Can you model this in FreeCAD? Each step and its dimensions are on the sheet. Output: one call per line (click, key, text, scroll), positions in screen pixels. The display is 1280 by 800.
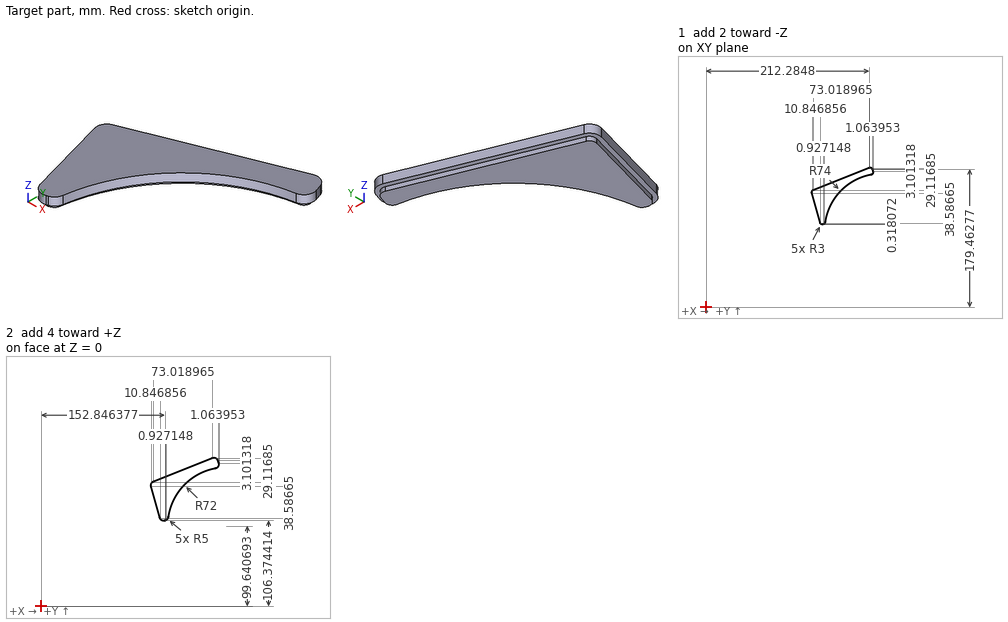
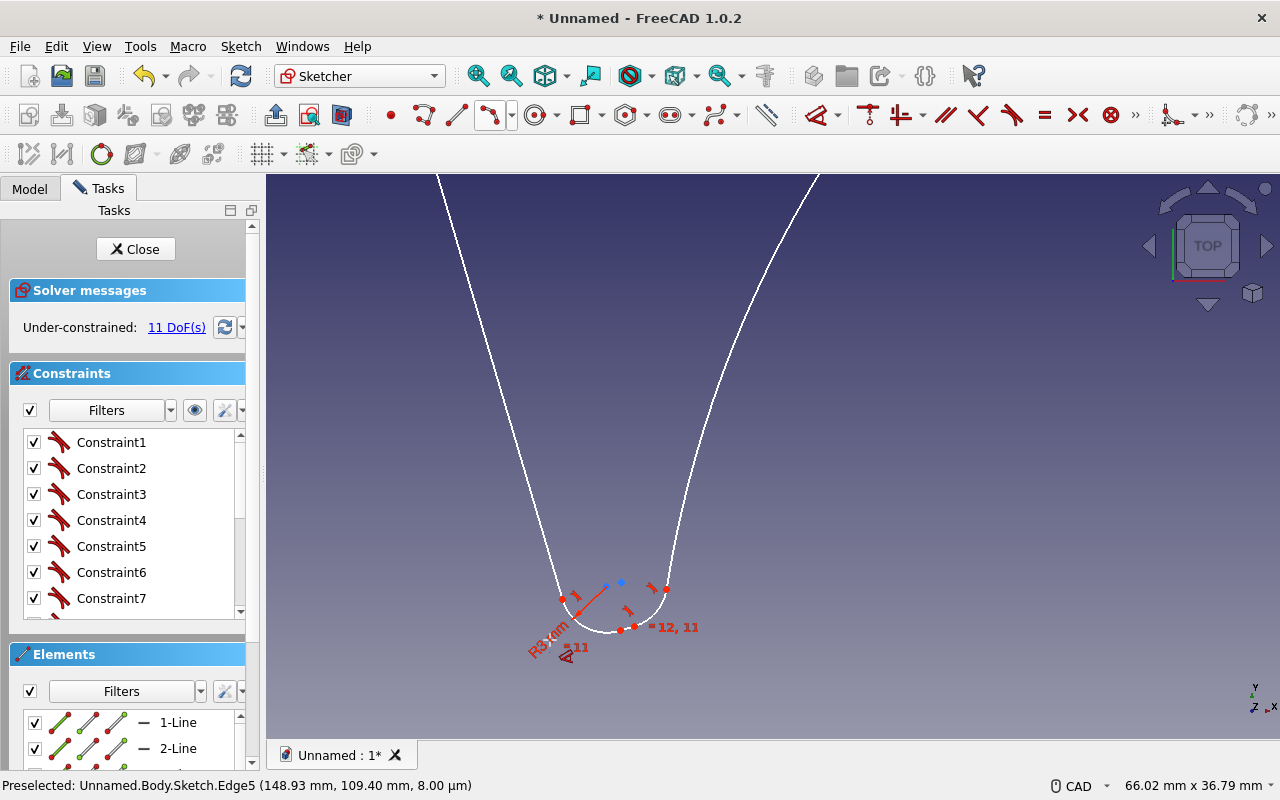
click(744, 321)
click(715, 308)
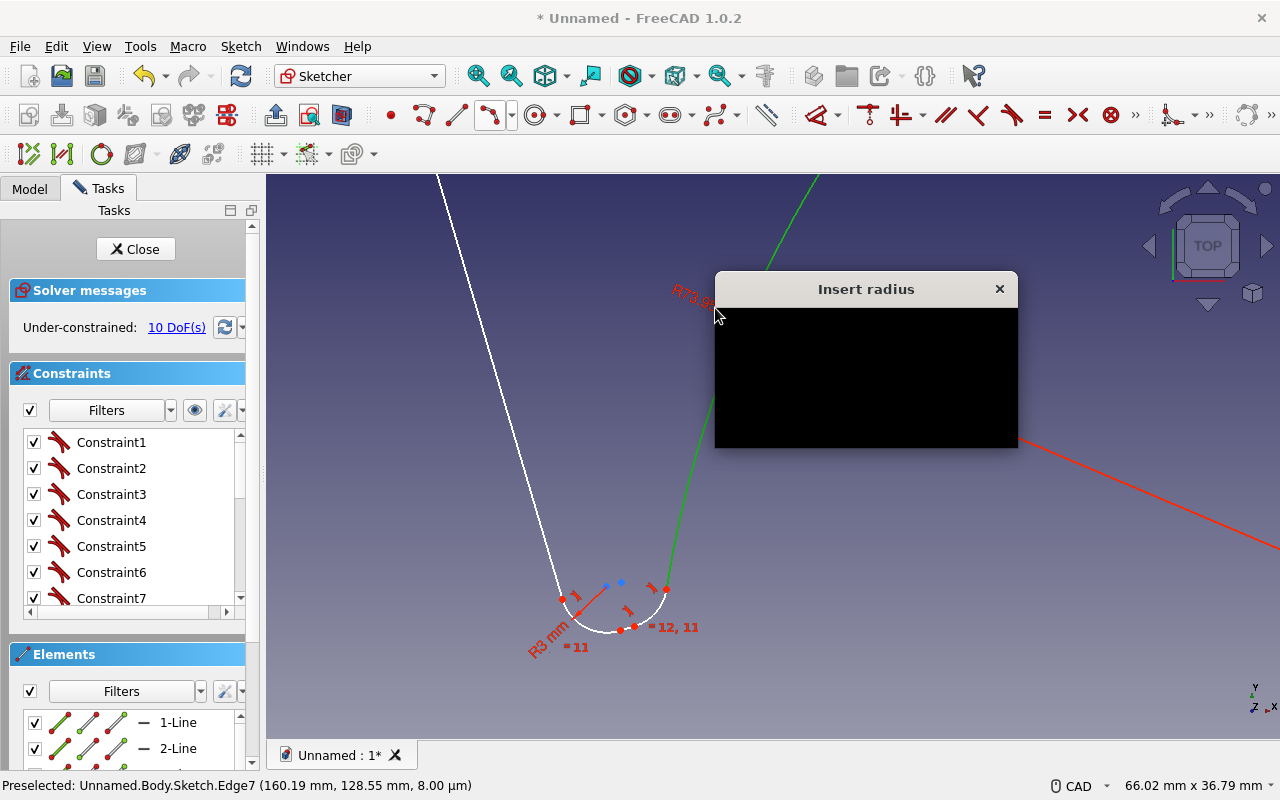
text(74)
key(Return)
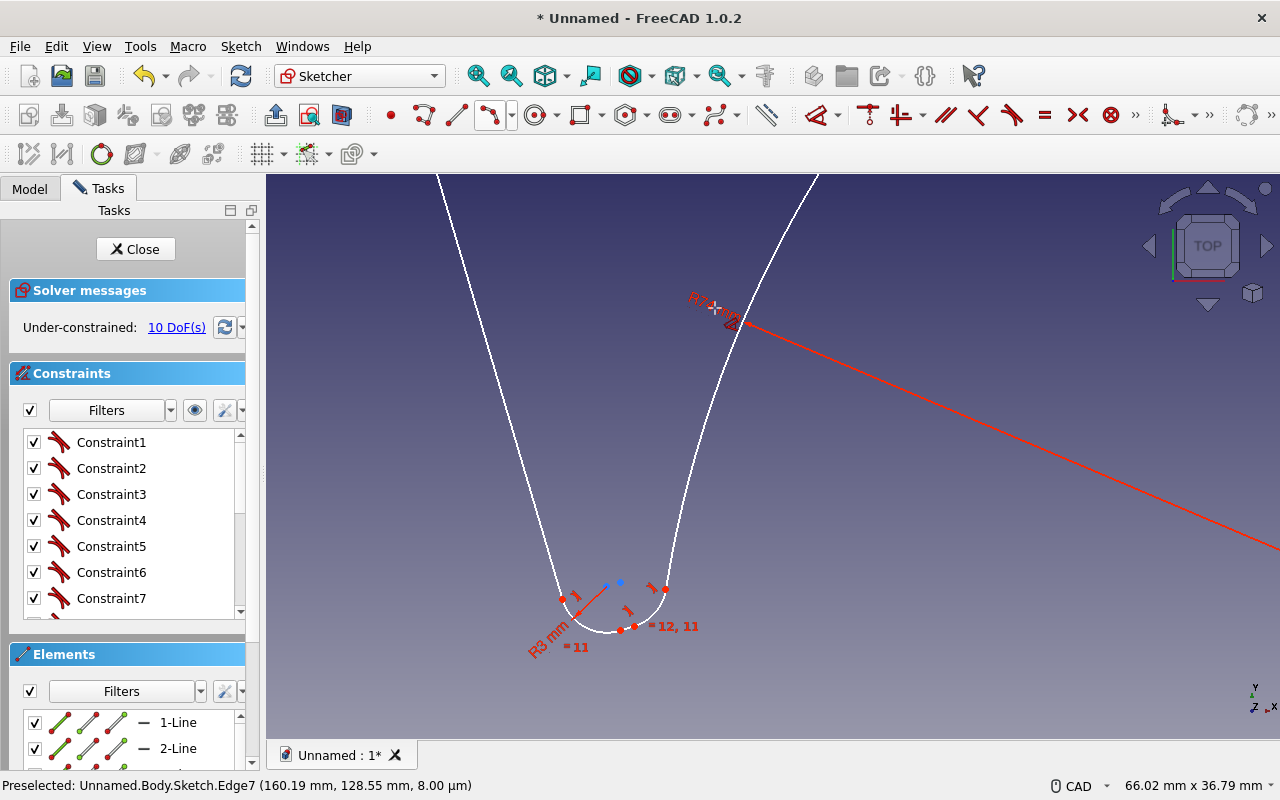
scroll(574, 621, down, 6)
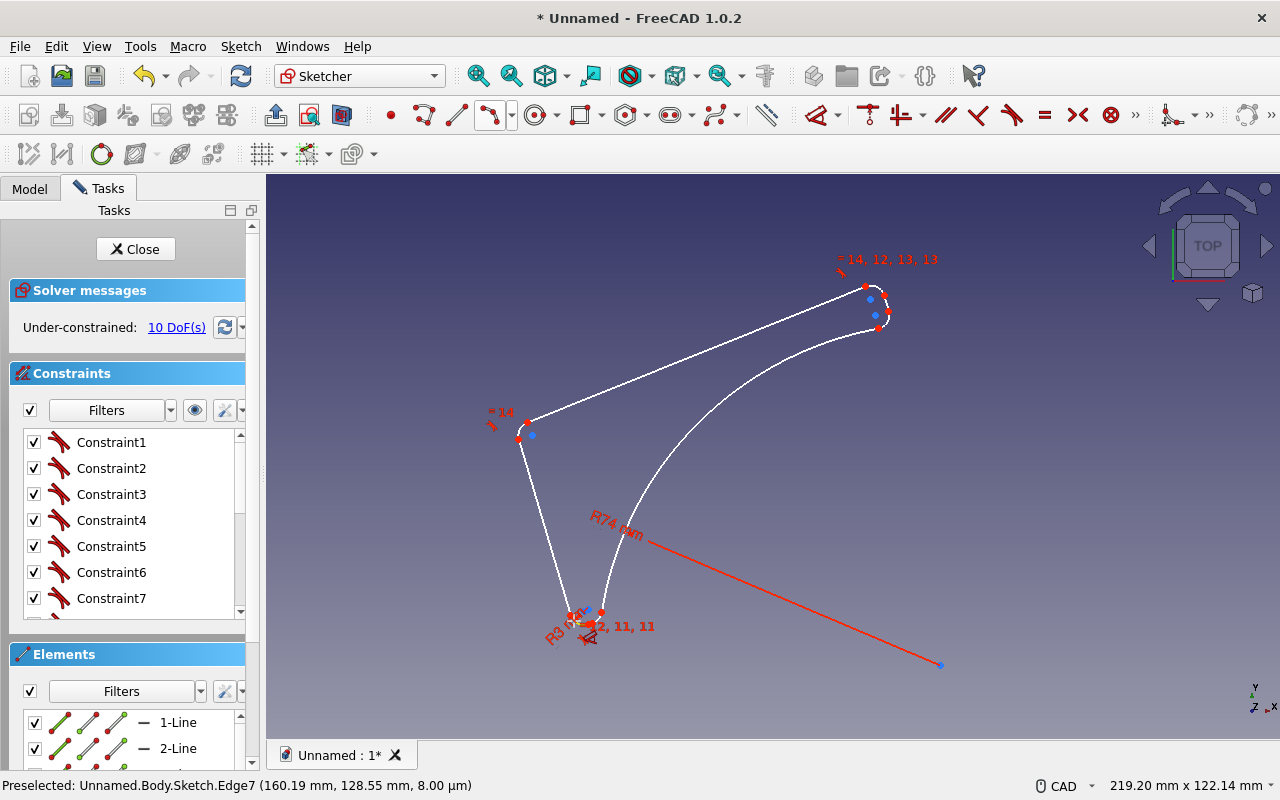
click(866, 287)
click(580, 253)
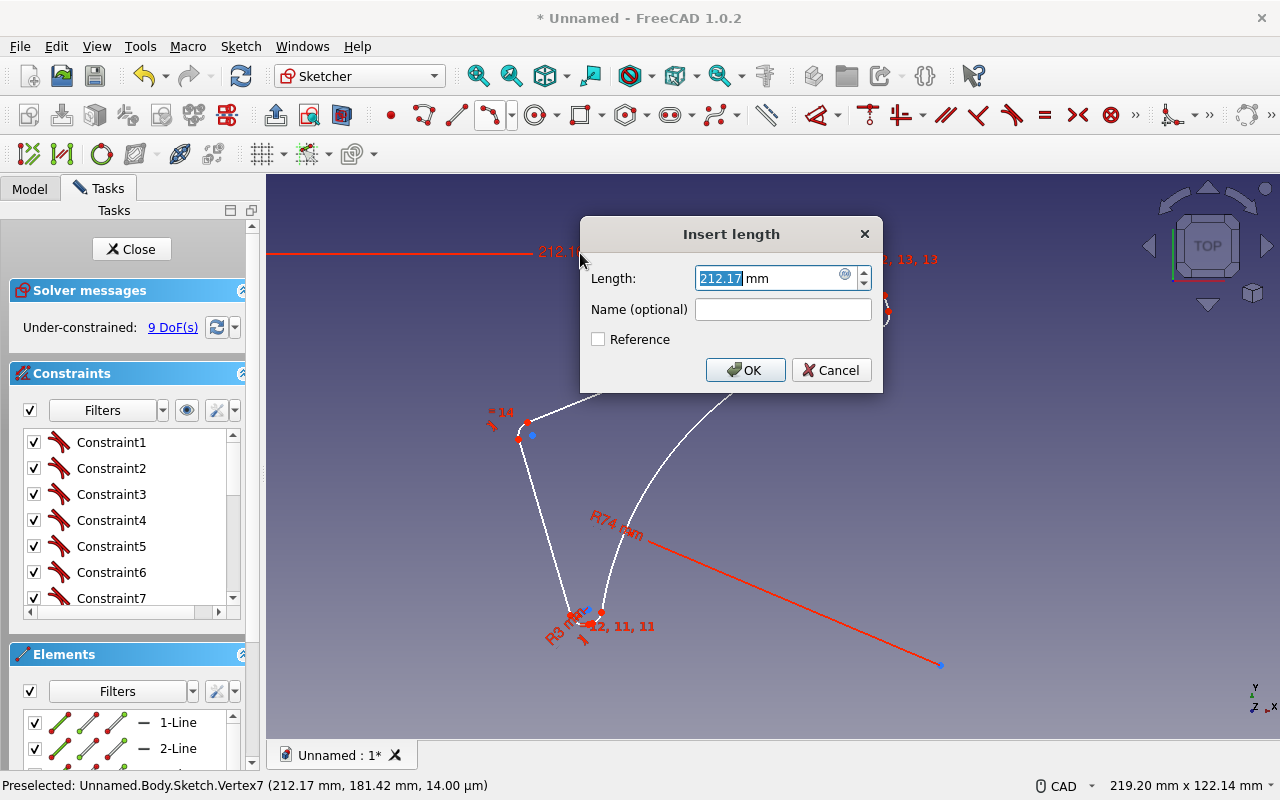
text(212.2848)
key(Return)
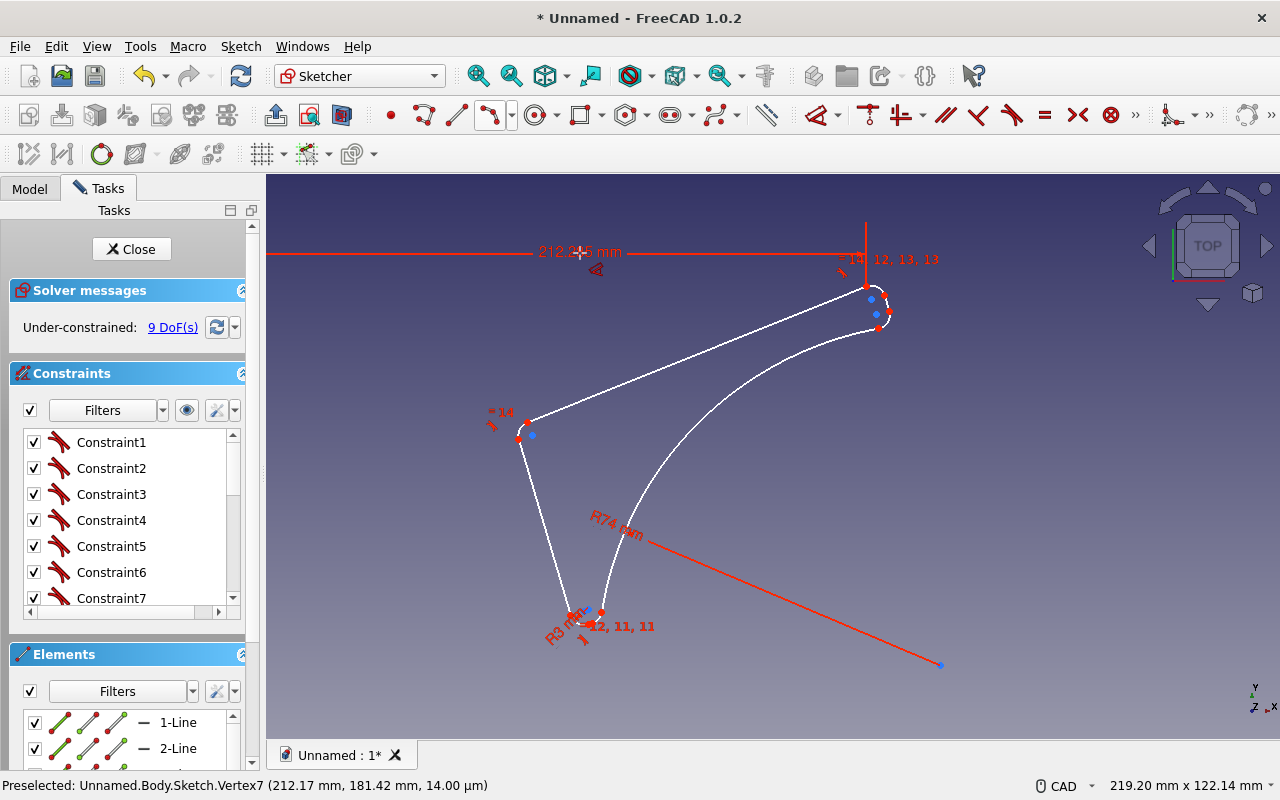
click(535, 492)
click(485, 527)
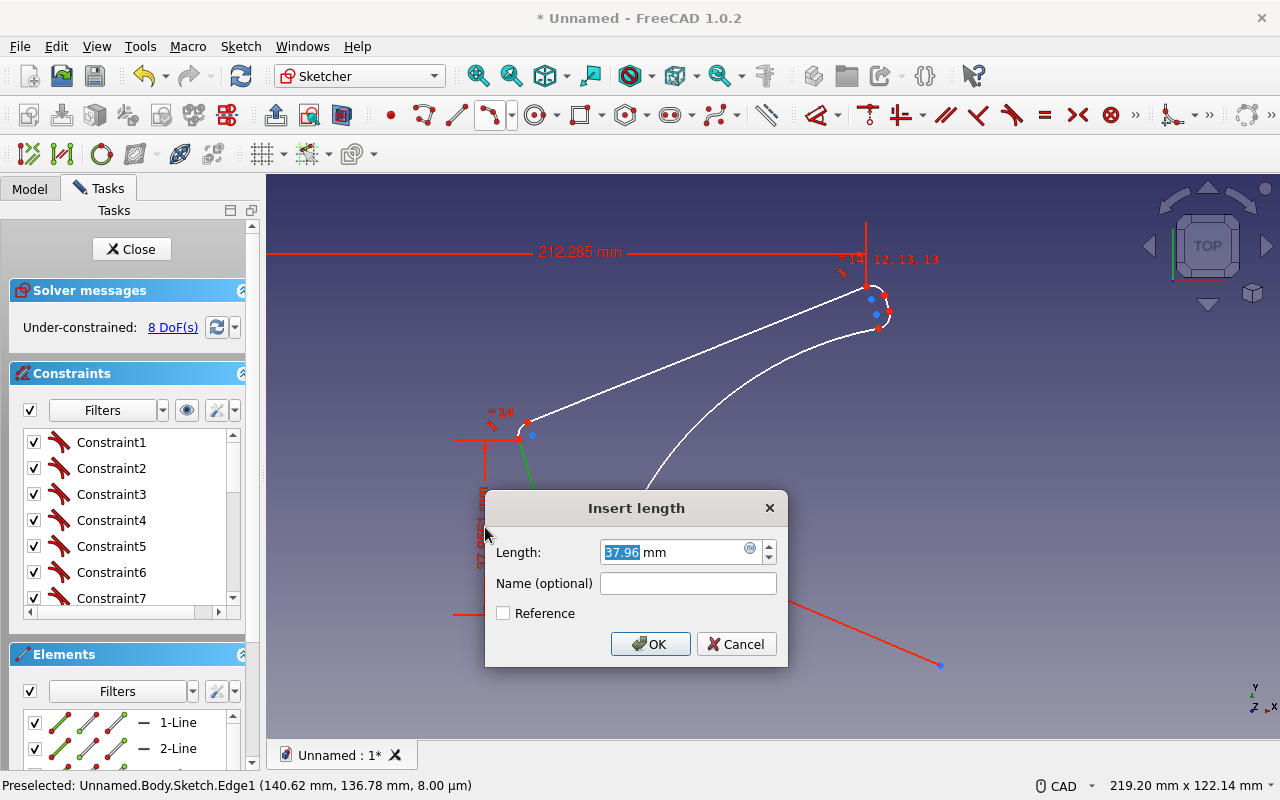
text(38.58665)
key(Return)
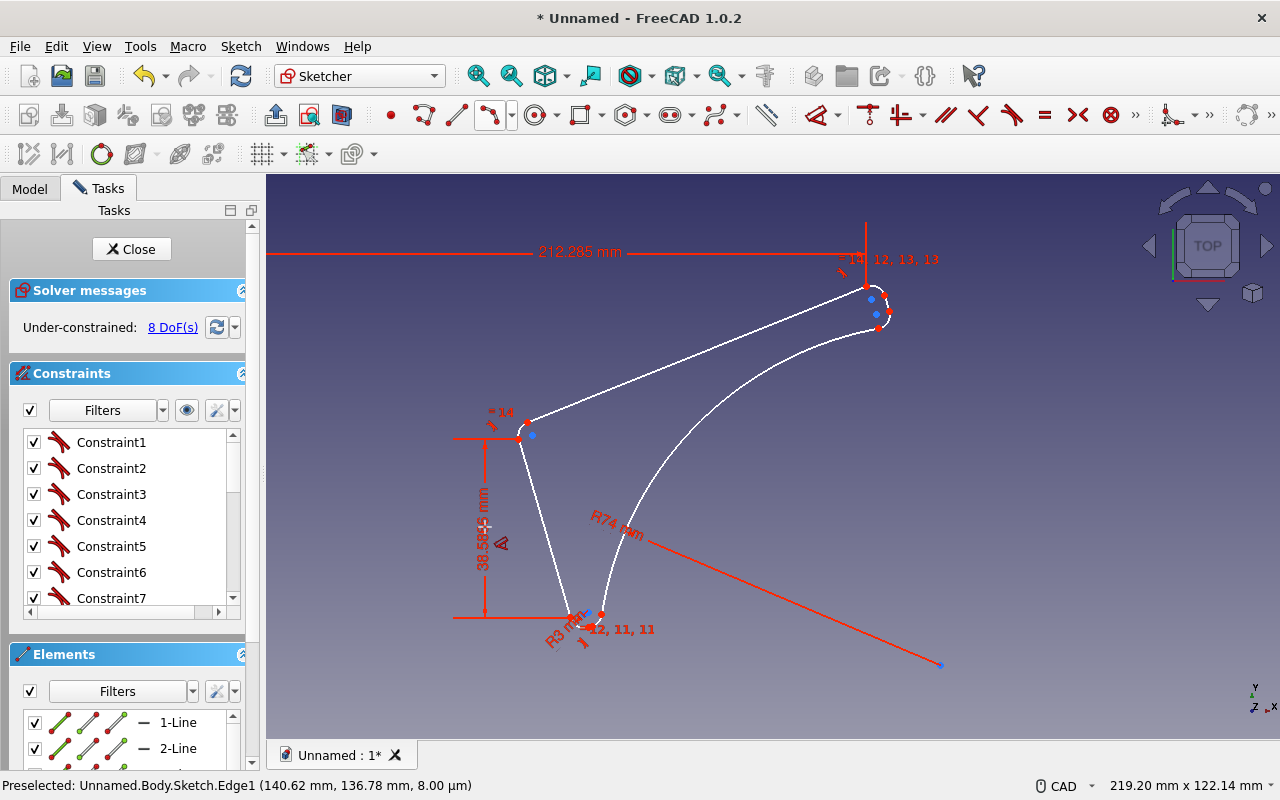
scroll(590, 627, up, 12)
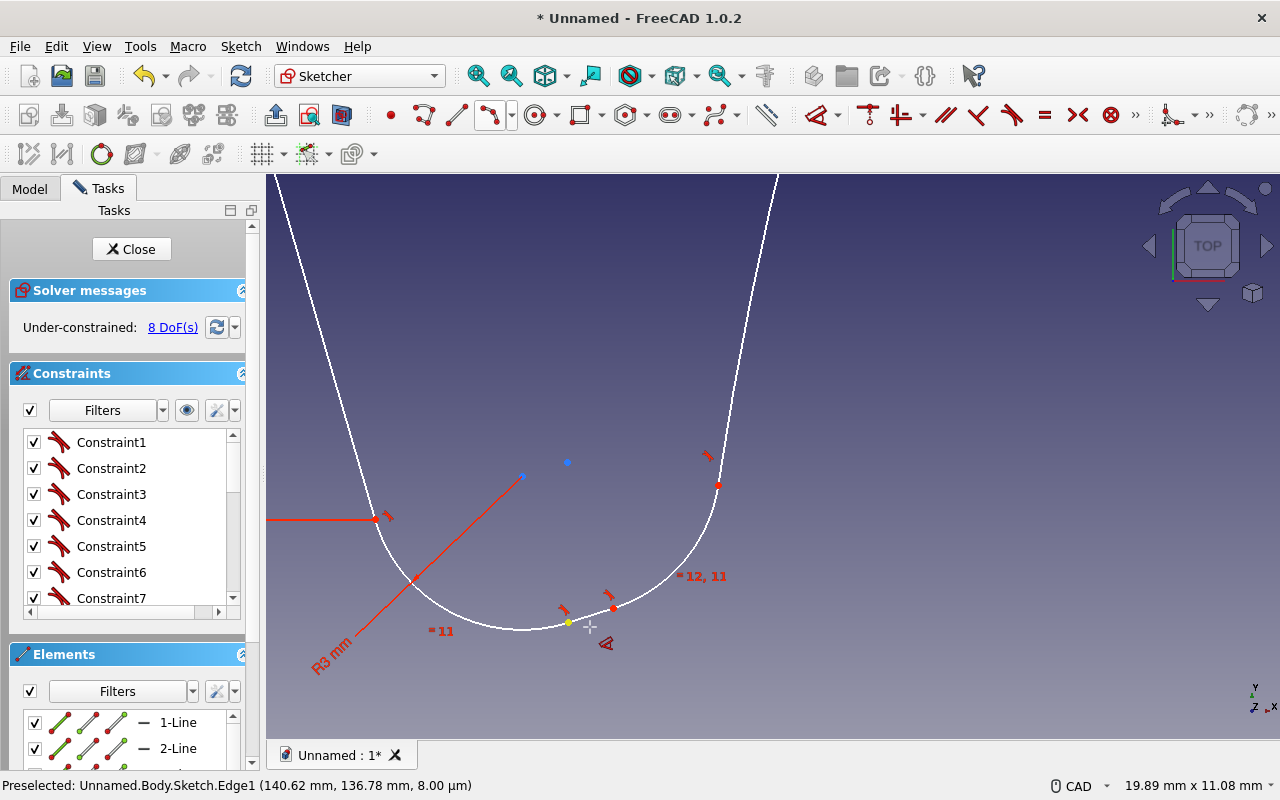
click(591, 615)
click(591, 657)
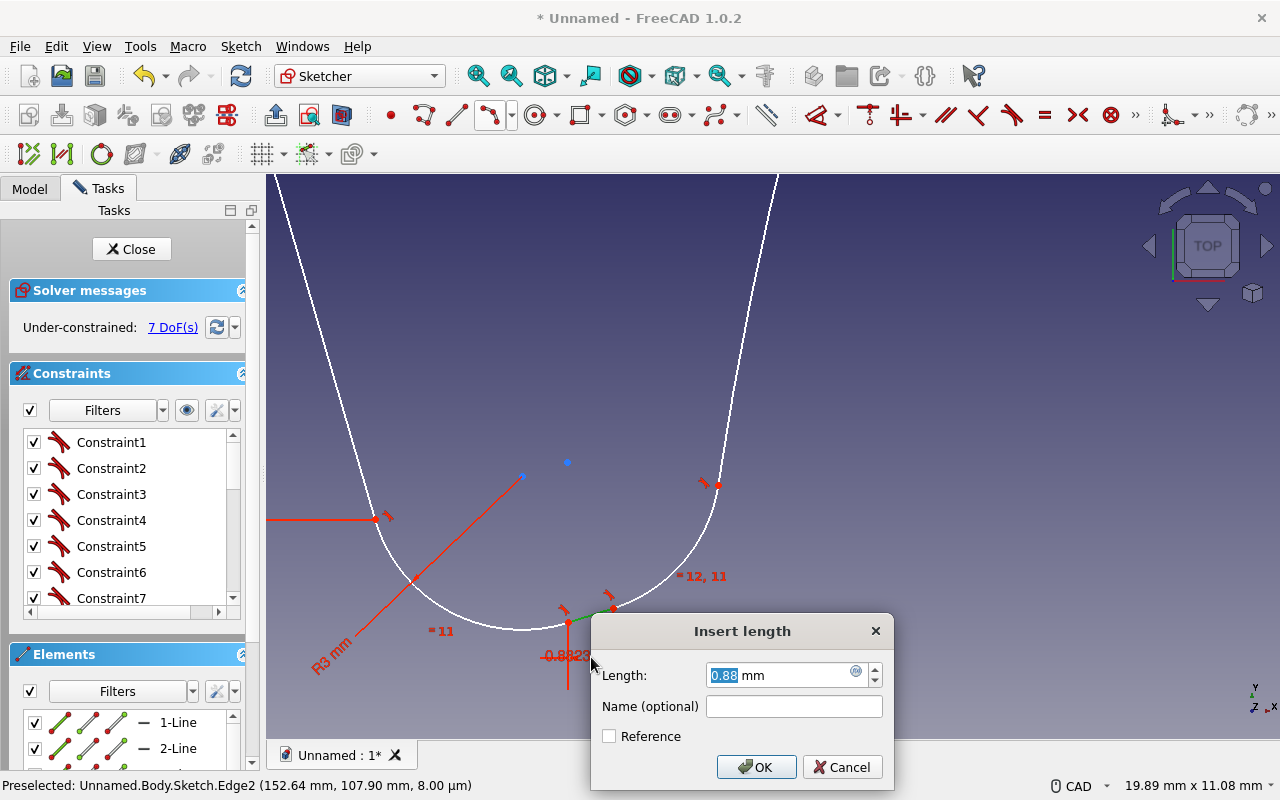
text(0.927148)
key(Return)